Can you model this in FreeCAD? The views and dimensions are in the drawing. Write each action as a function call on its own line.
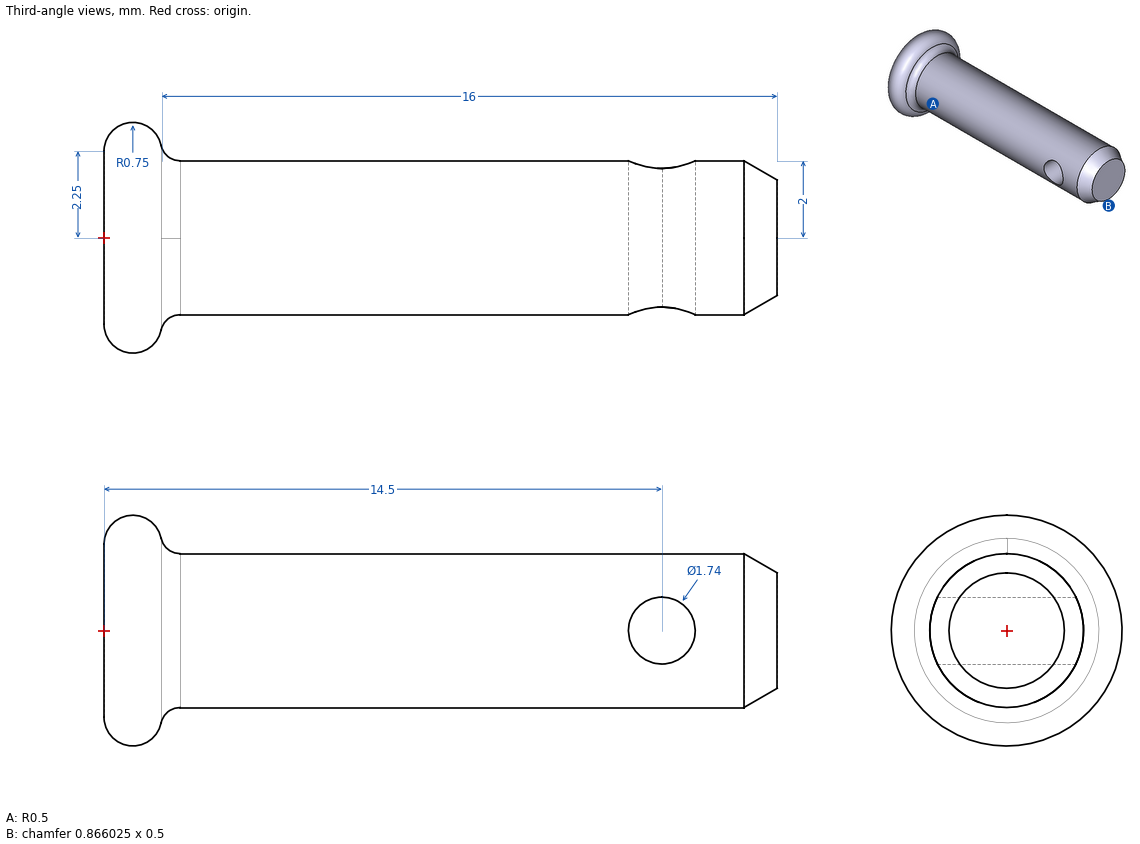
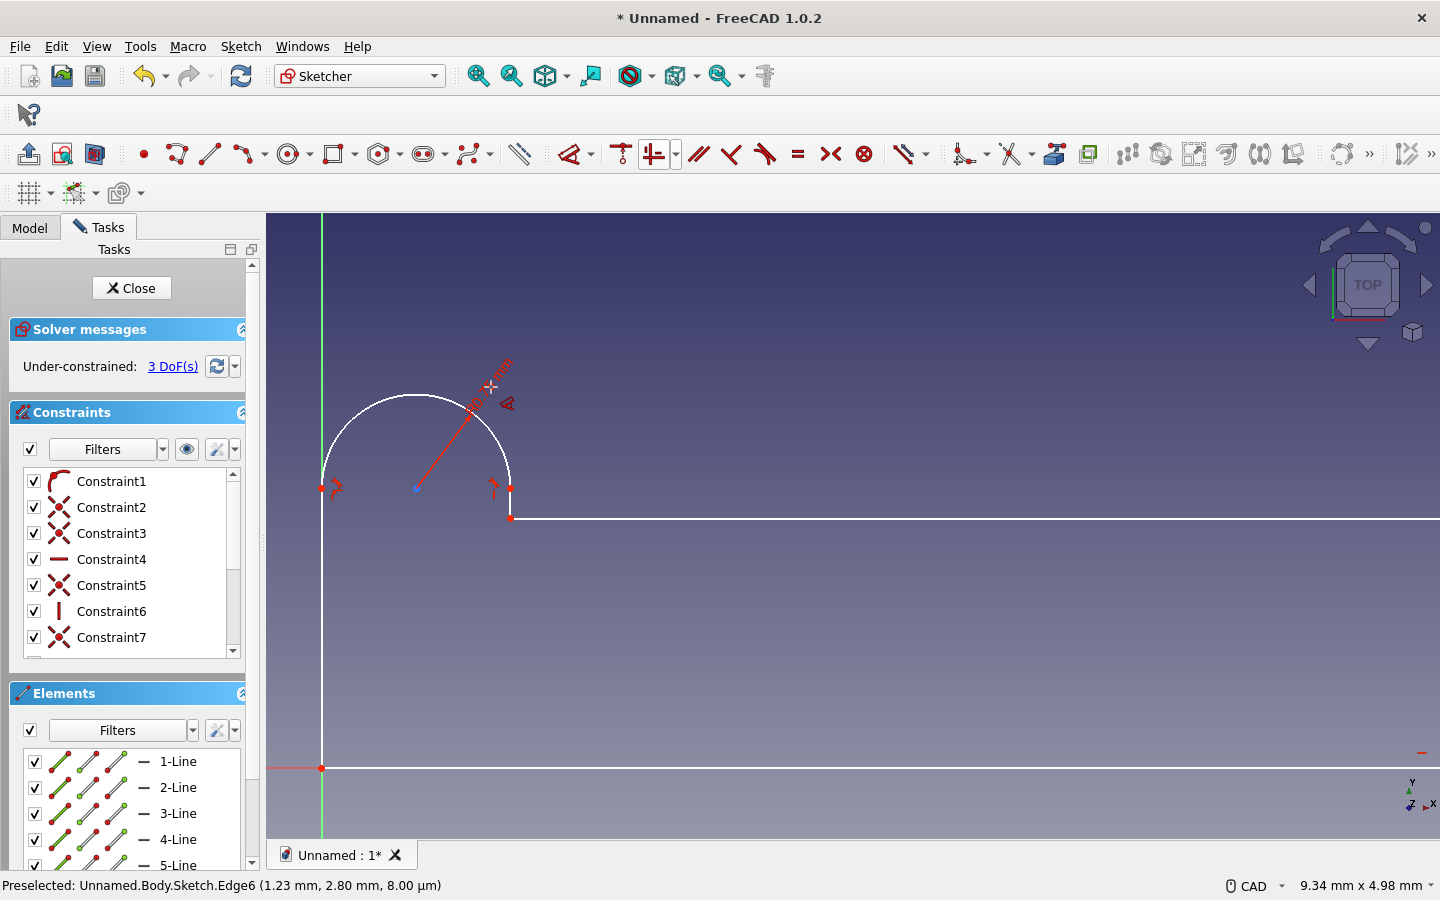
scroll(510, 503, down, 6)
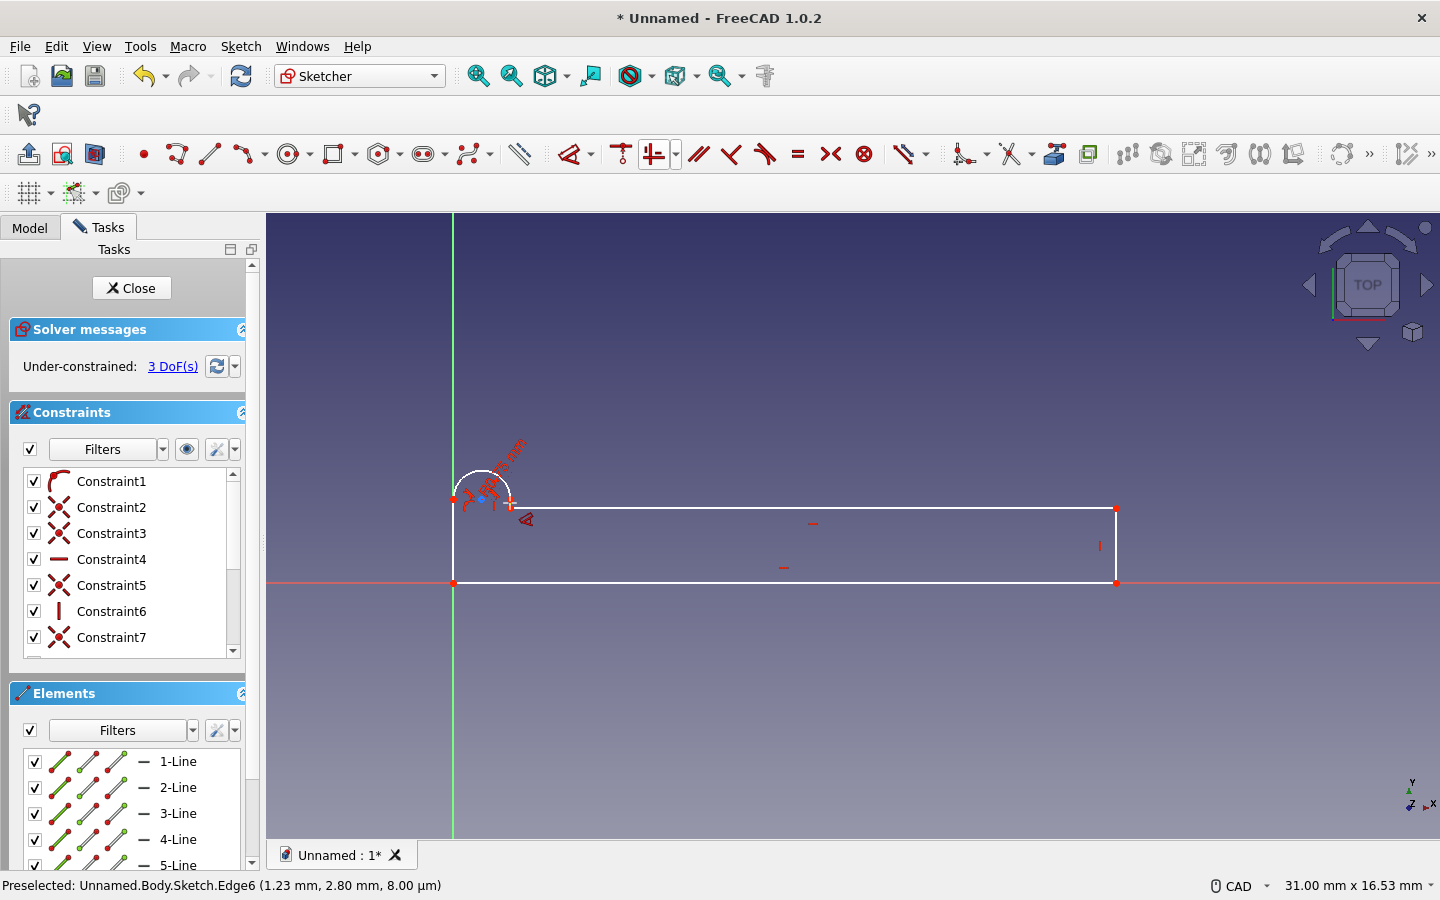
click(1116, 561)
click(1150, 546)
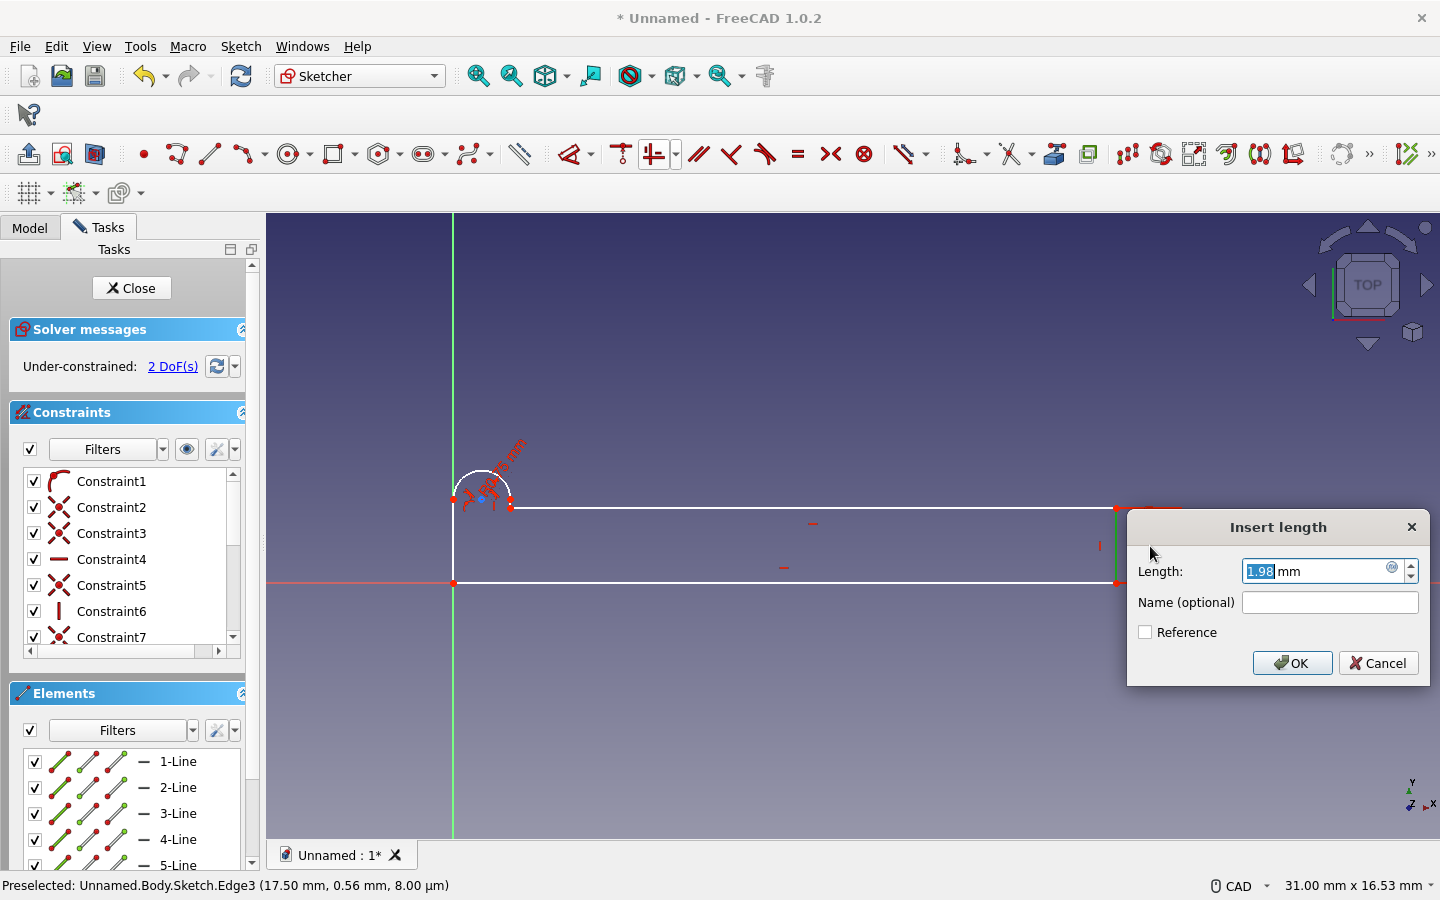
text(2)
key(Return)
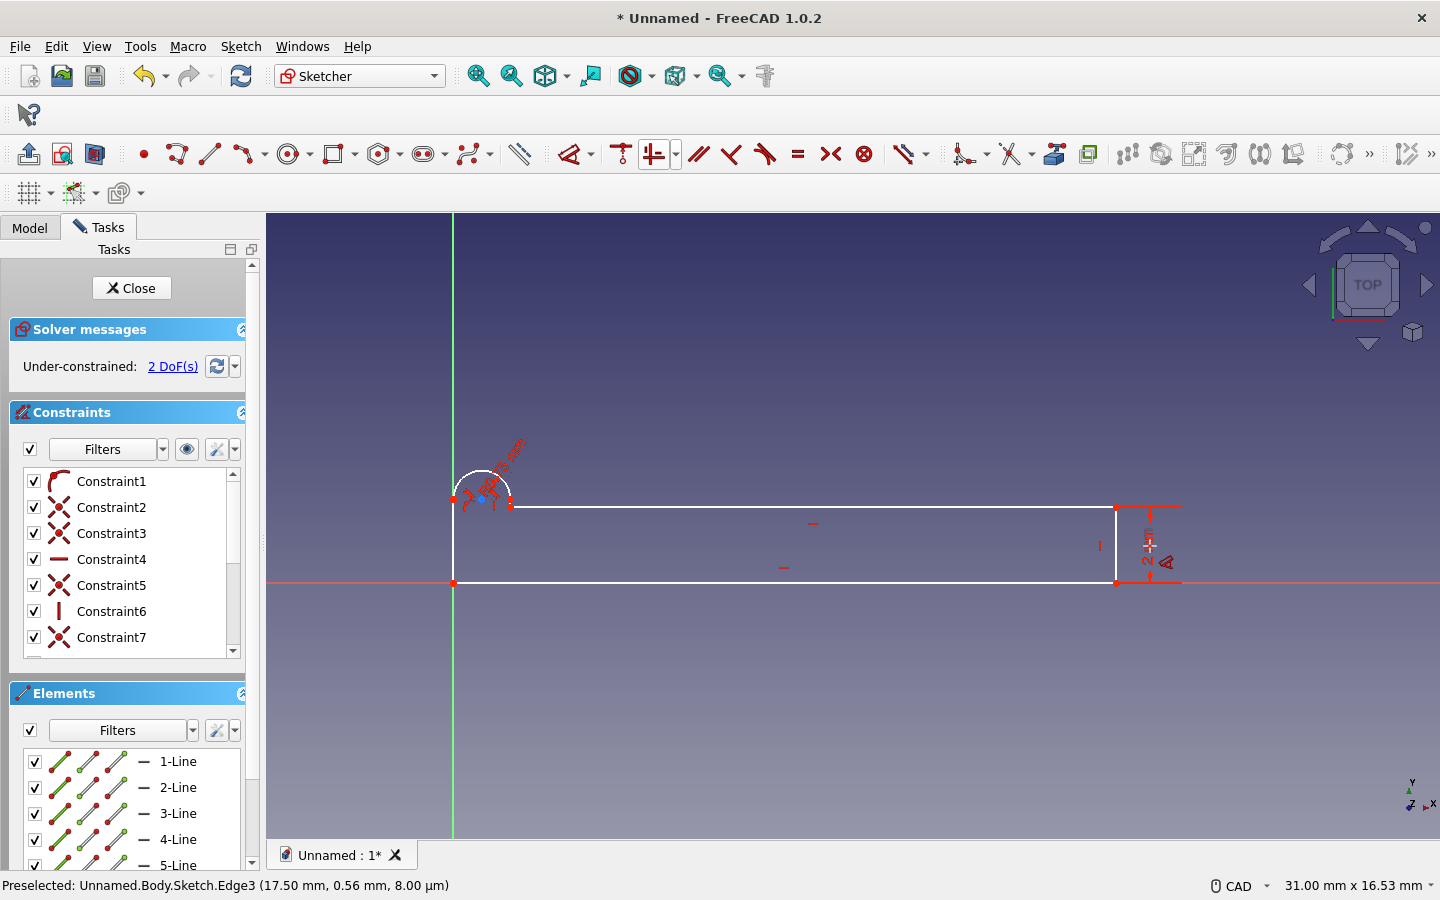
click(934, 507)
click(813, 473)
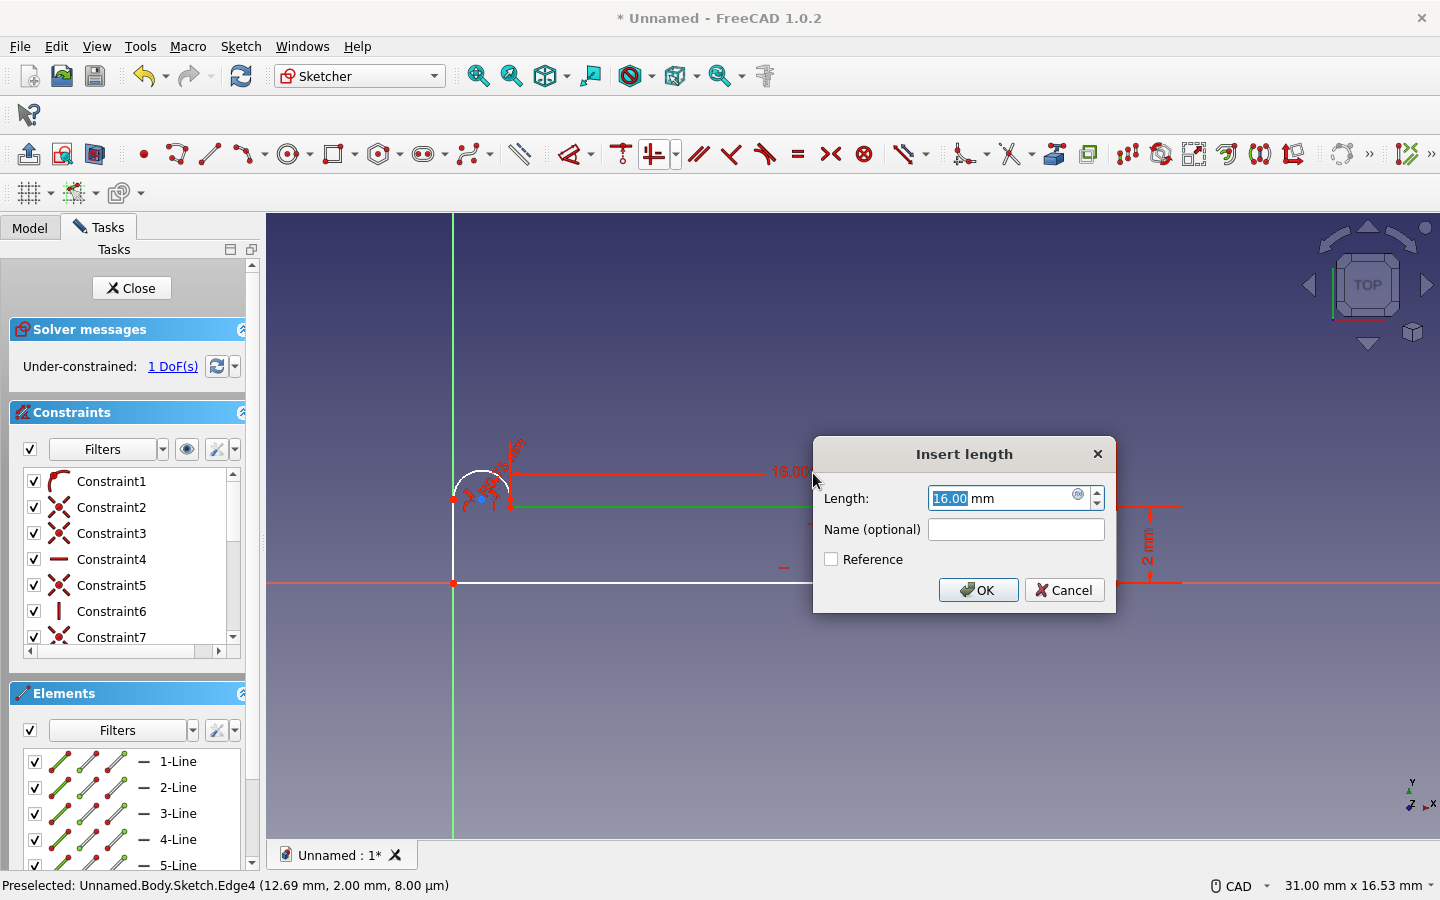
text(16)
key(Return)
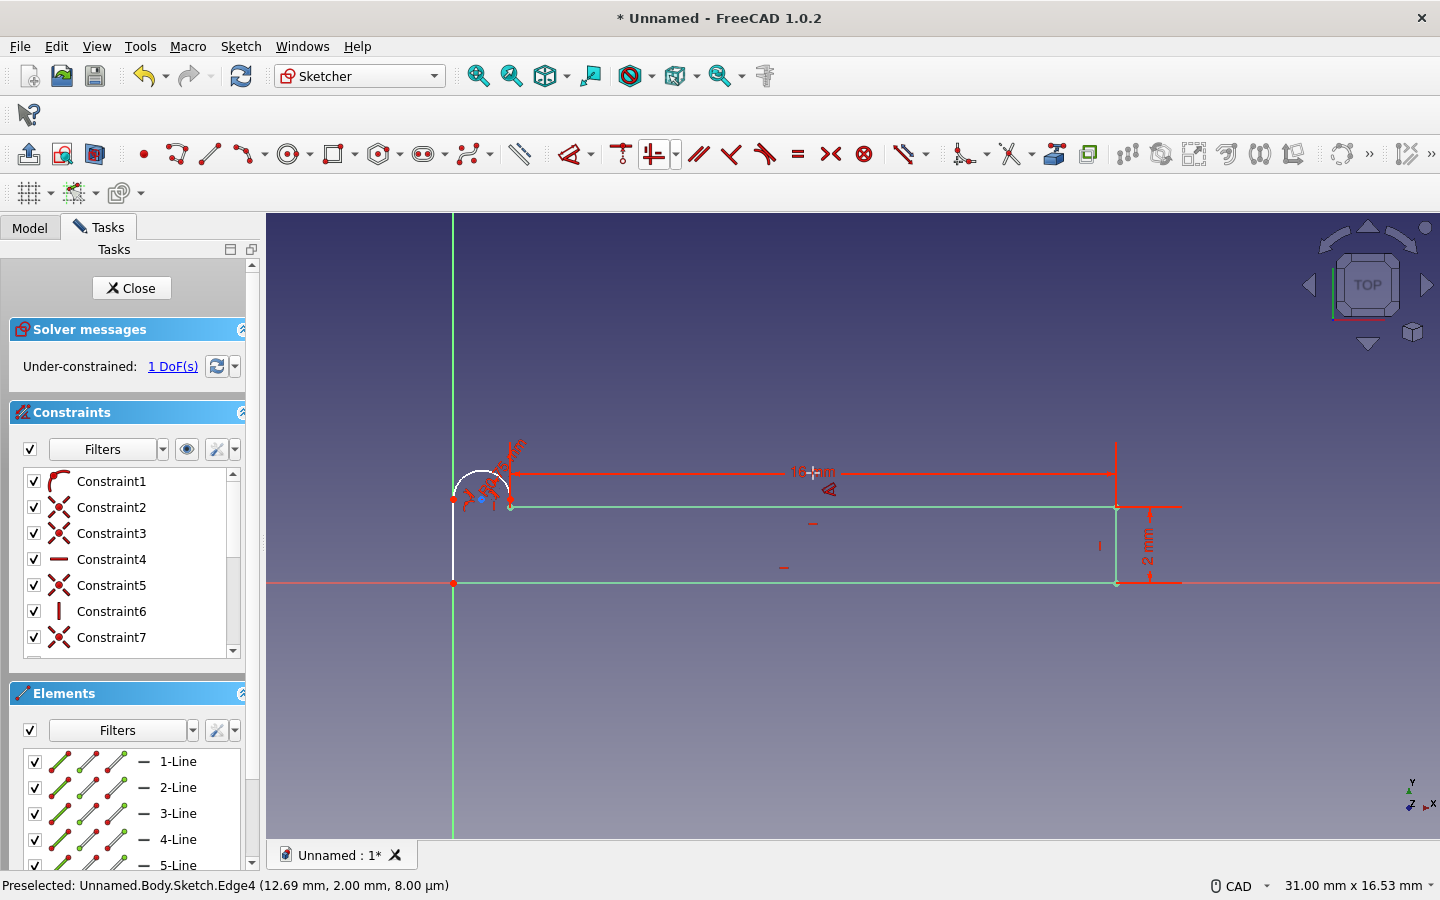
click(453, 524)
click(419, 541)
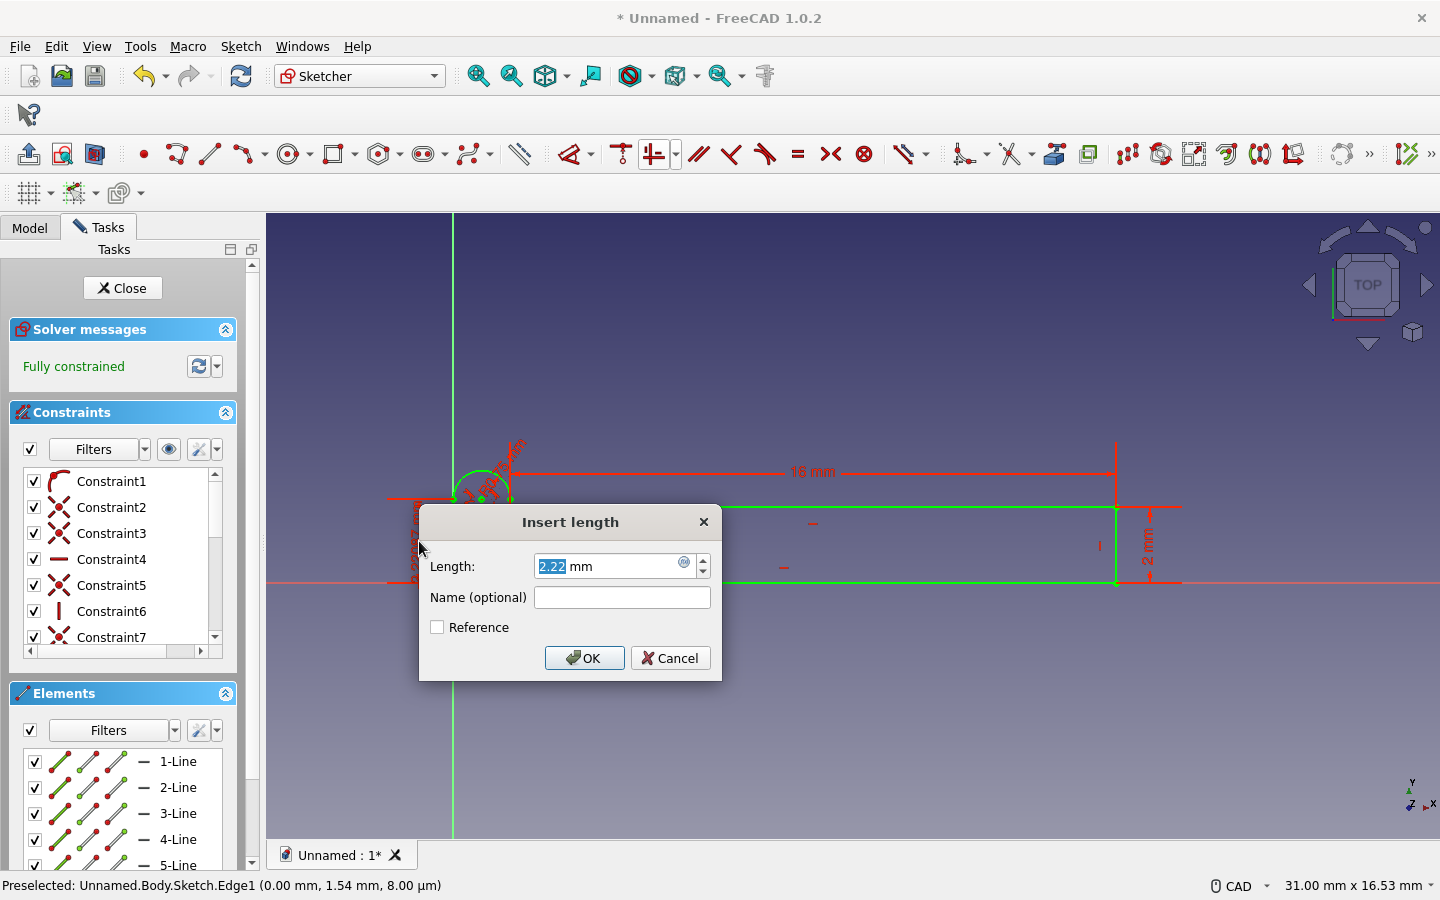
text(2.25)
key(Return)
key(Escape)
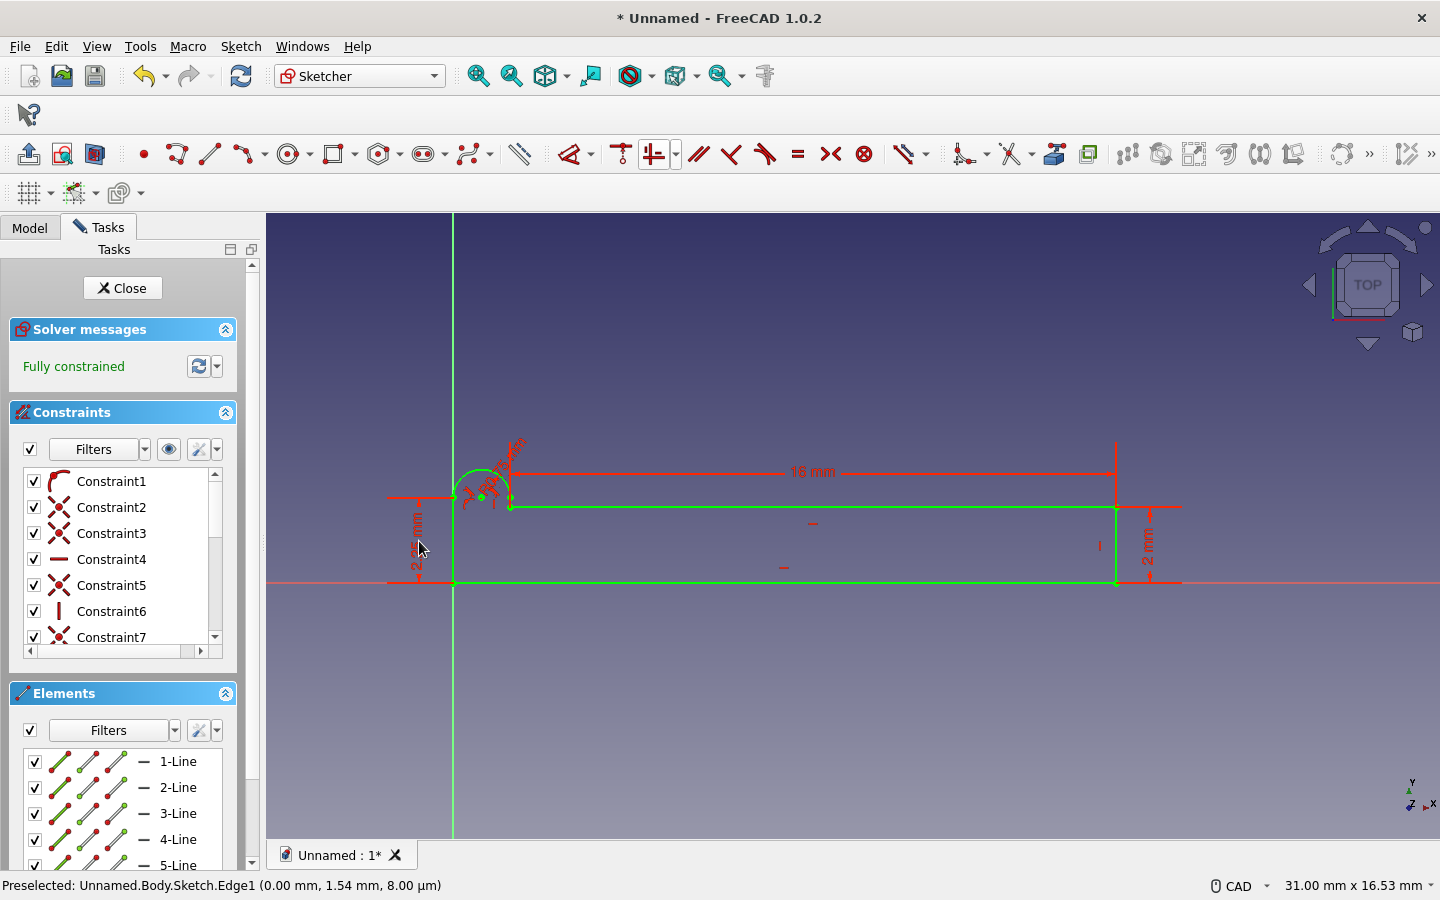
click(123, 288)